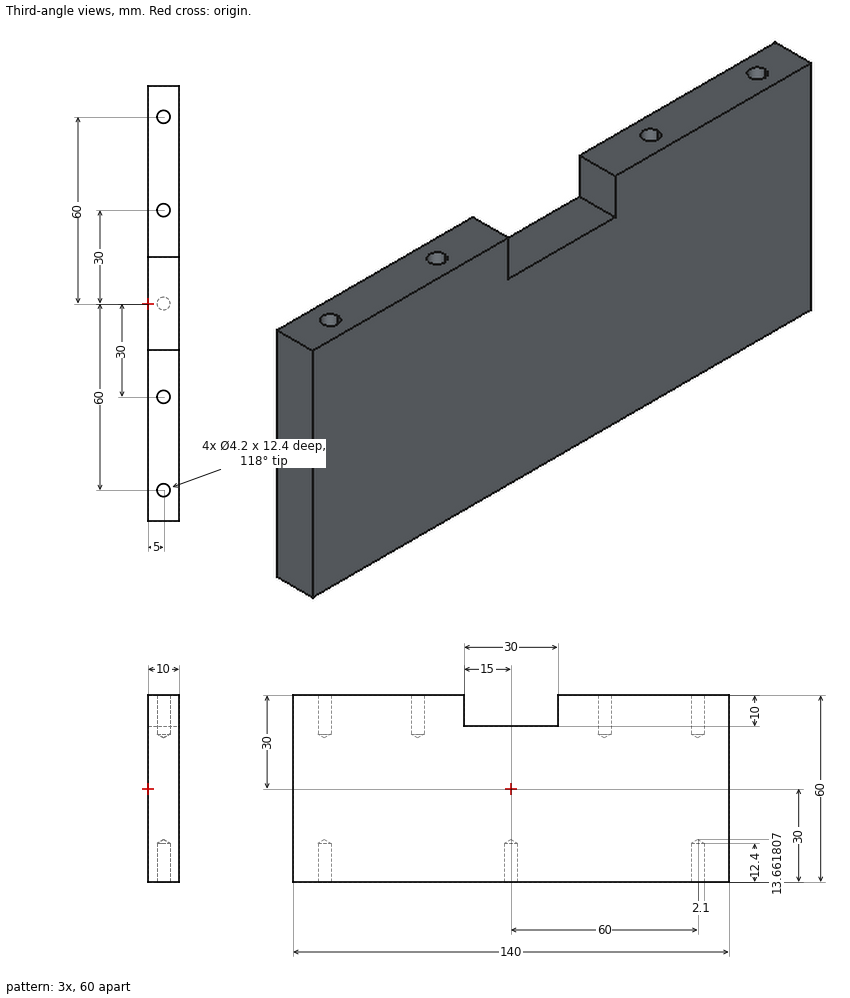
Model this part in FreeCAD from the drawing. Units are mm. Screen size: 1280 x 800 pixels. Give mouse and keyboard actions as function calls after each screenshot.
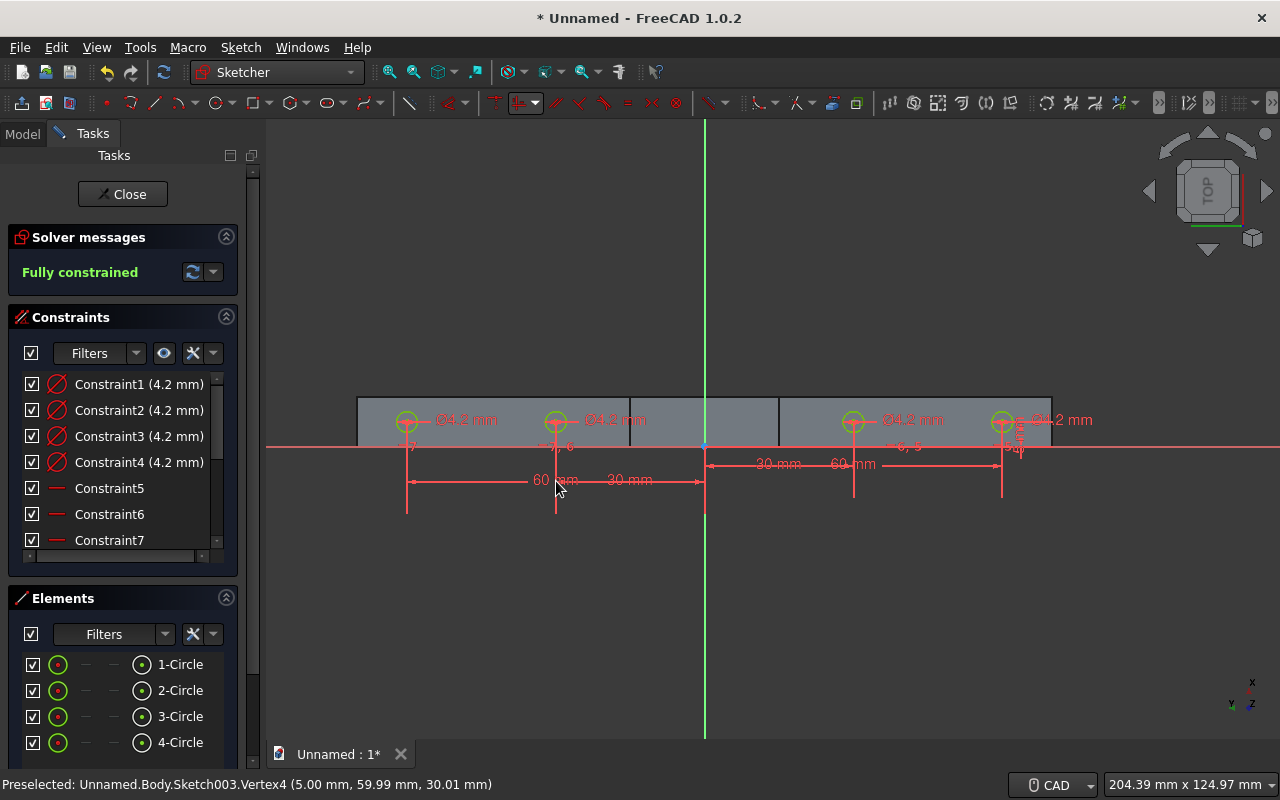
click(123, 194)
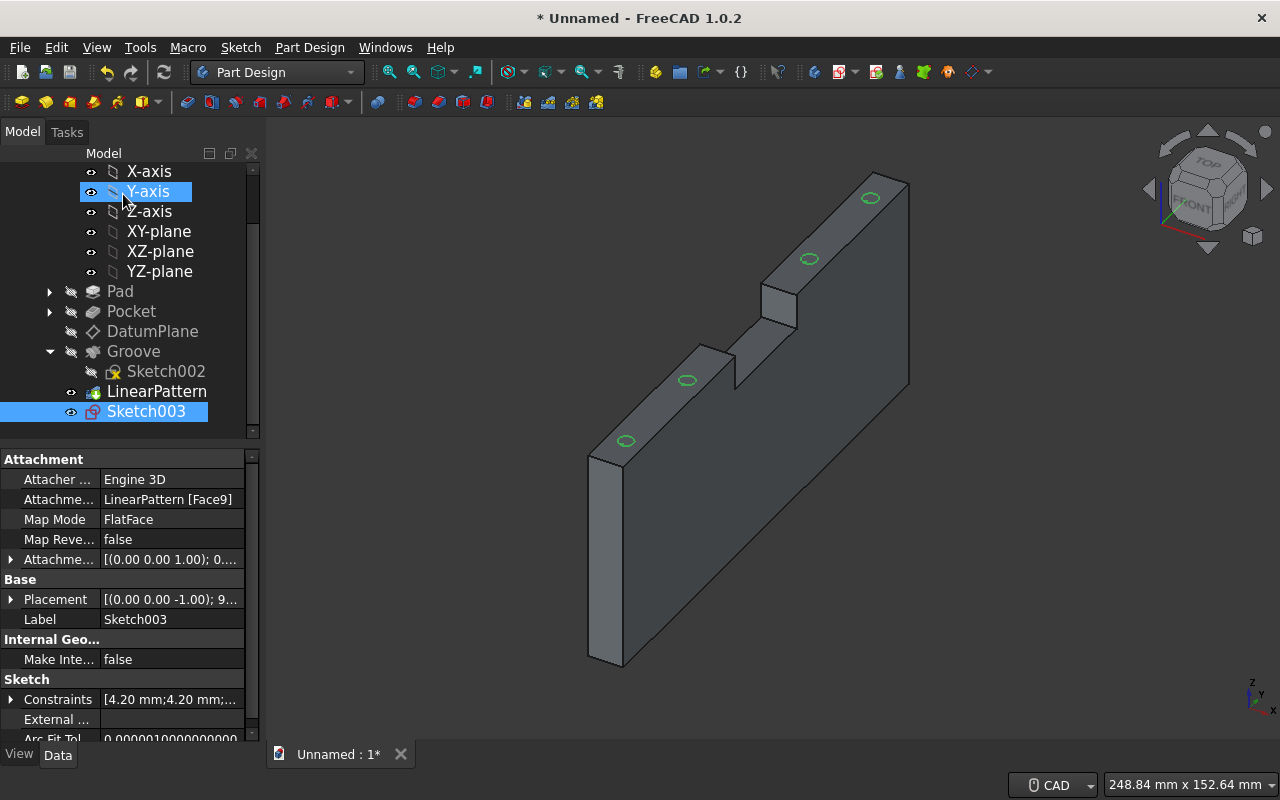
click(212, 102)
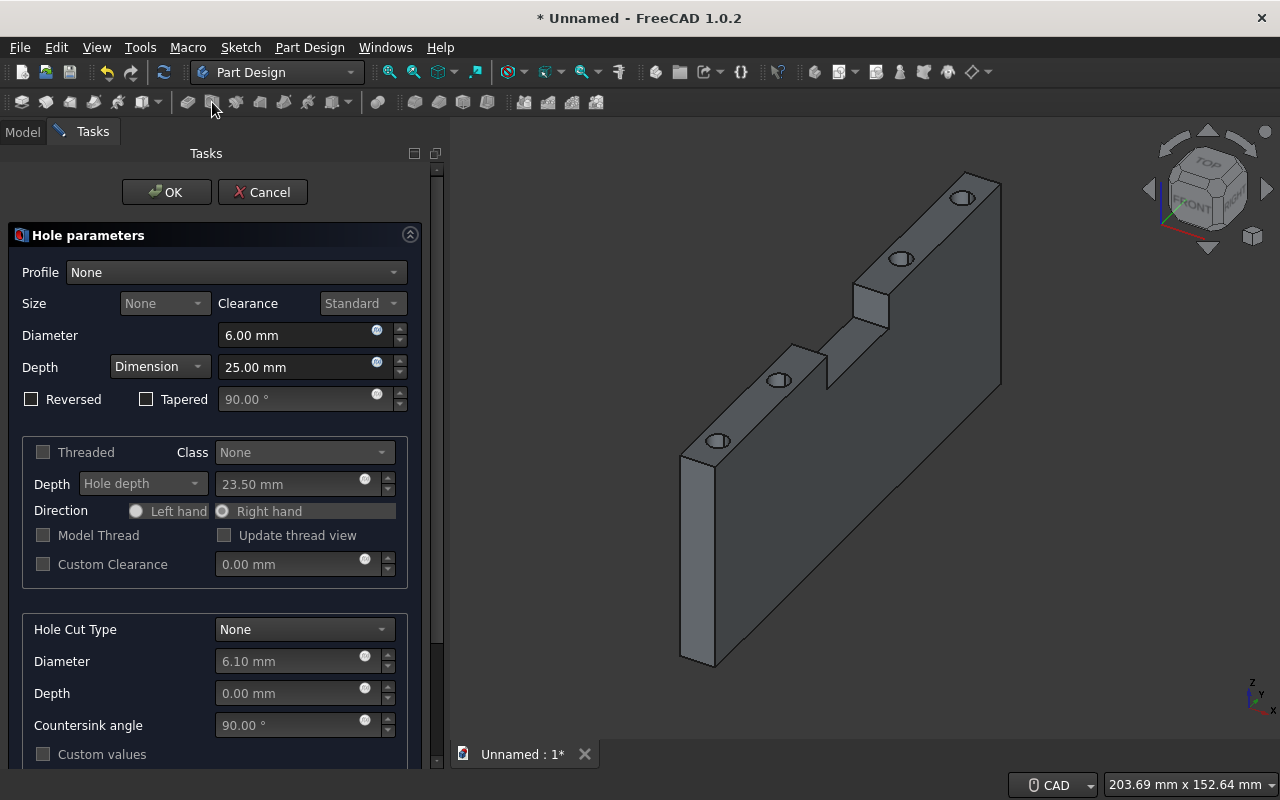
triple_click(305, 335)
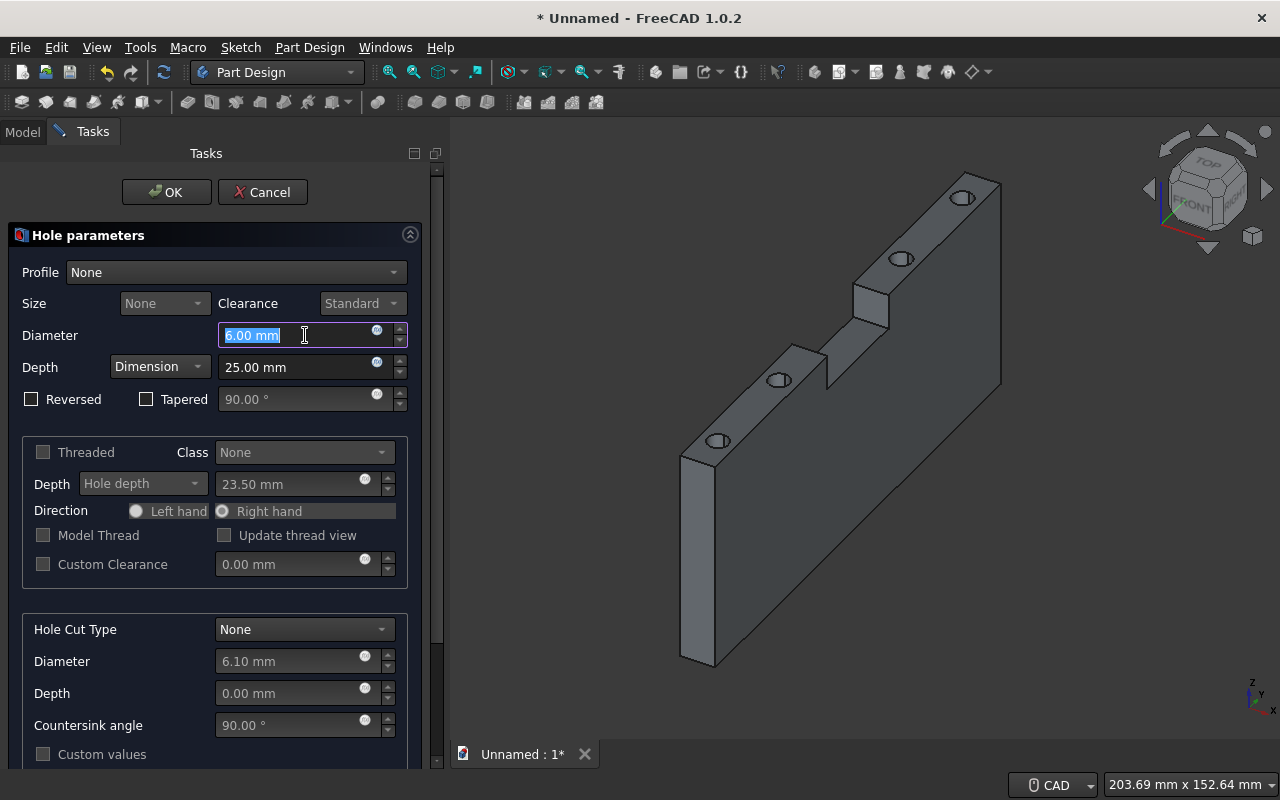
text(4.2)
key(Tab)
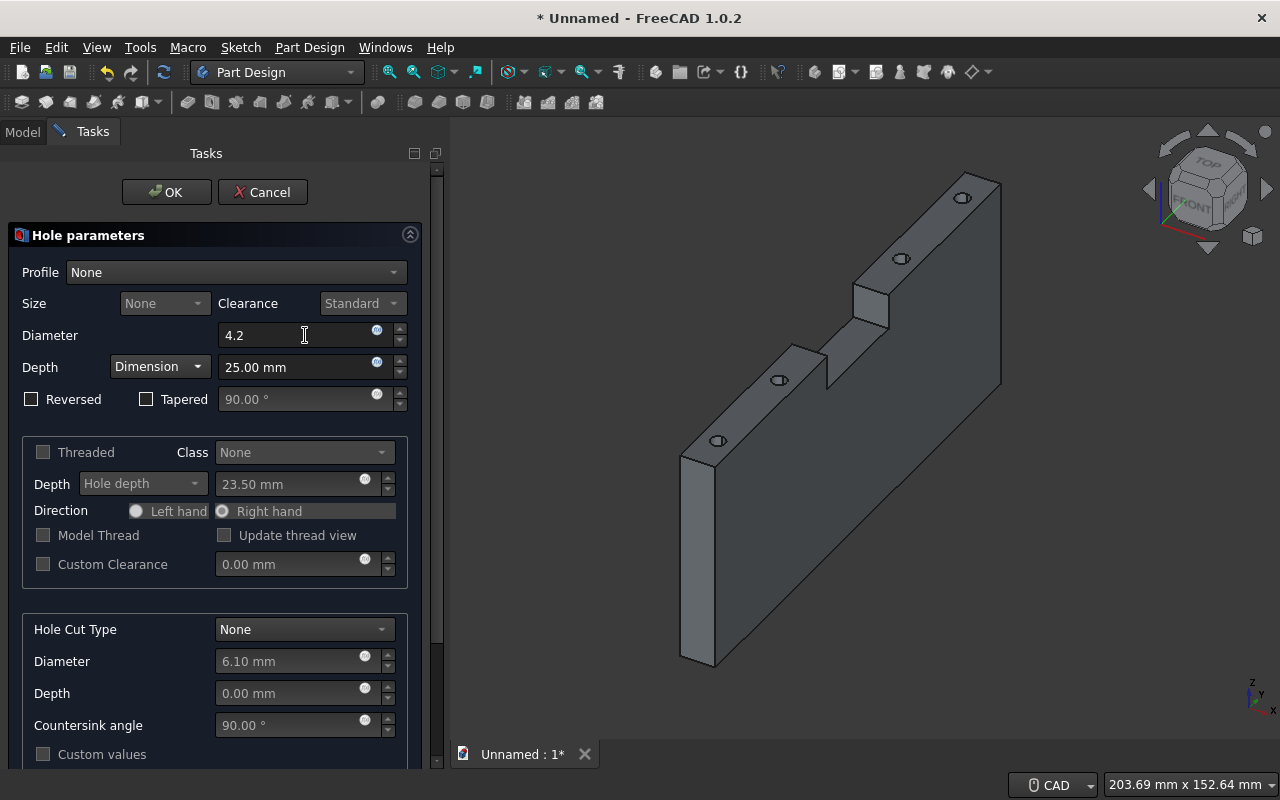
triple_click(305, 367)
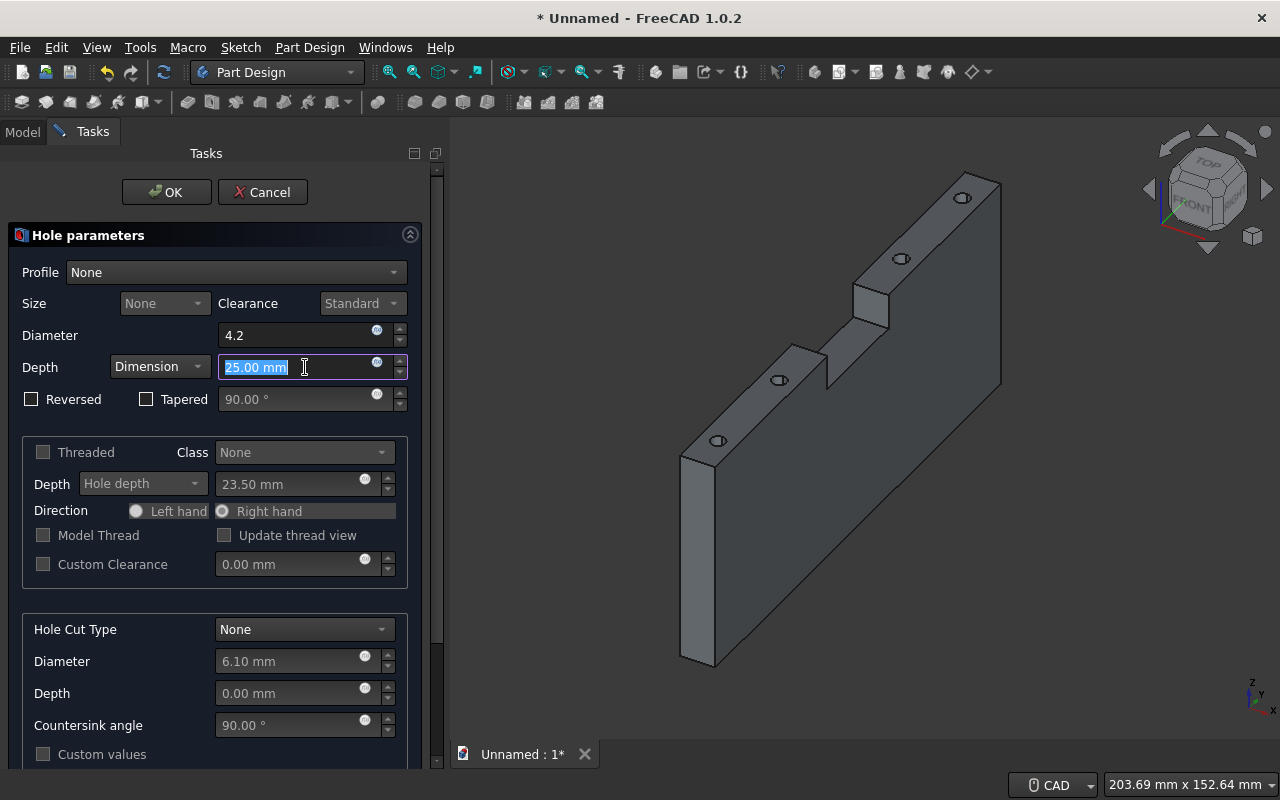
text(12.4)
key(Tab)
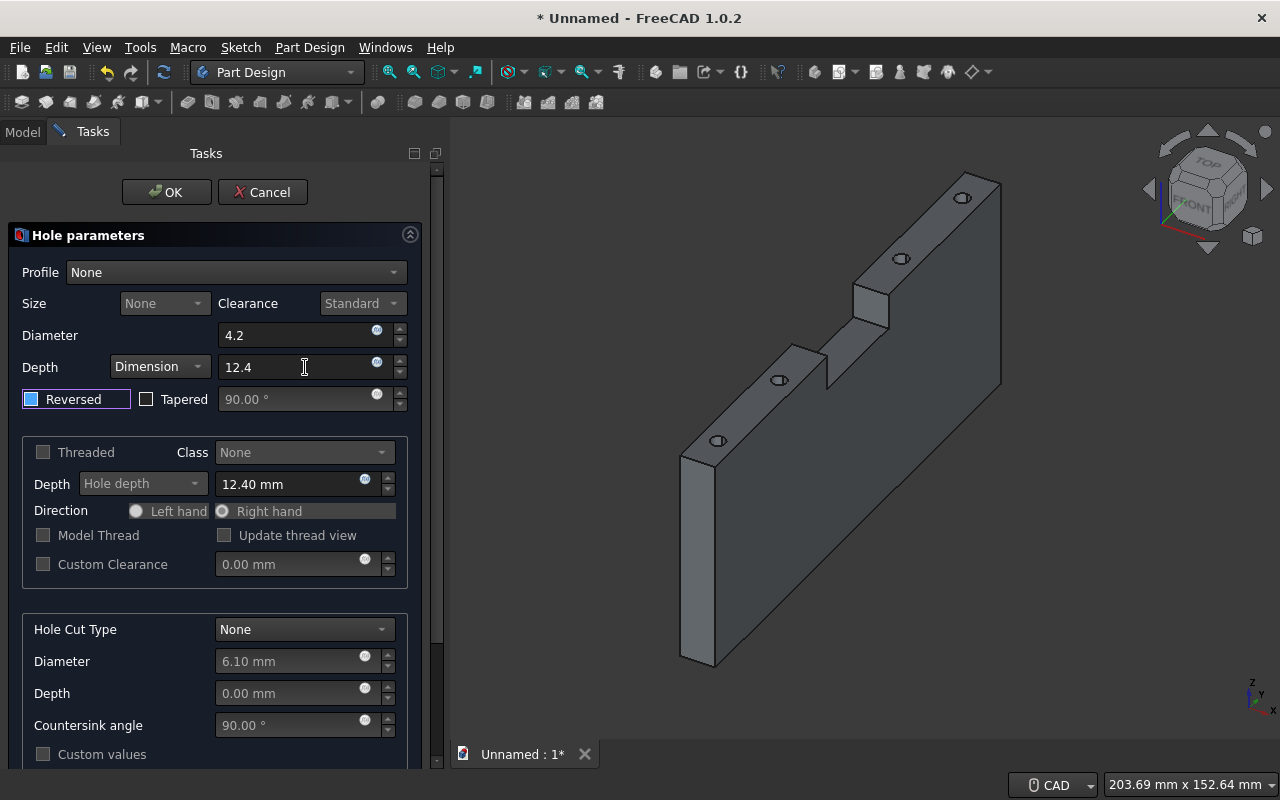
click(167, 192)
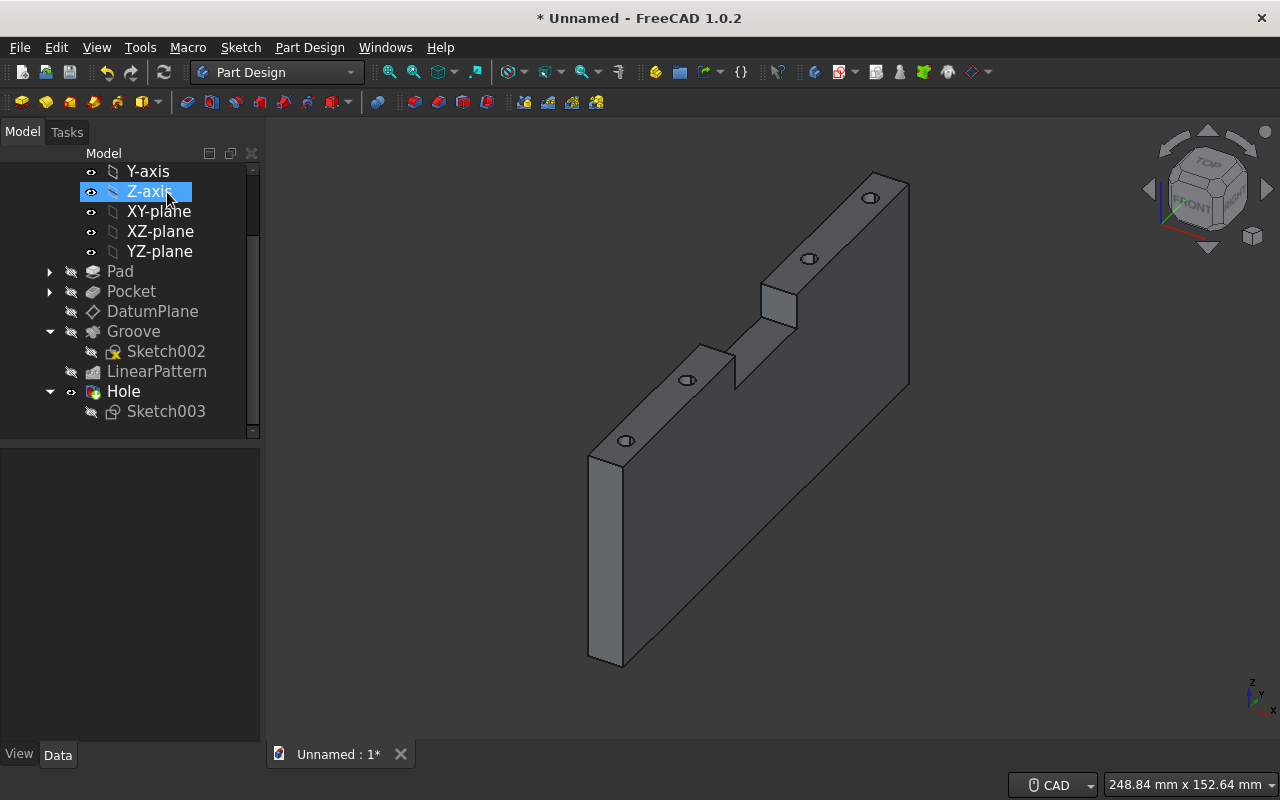
key(0)